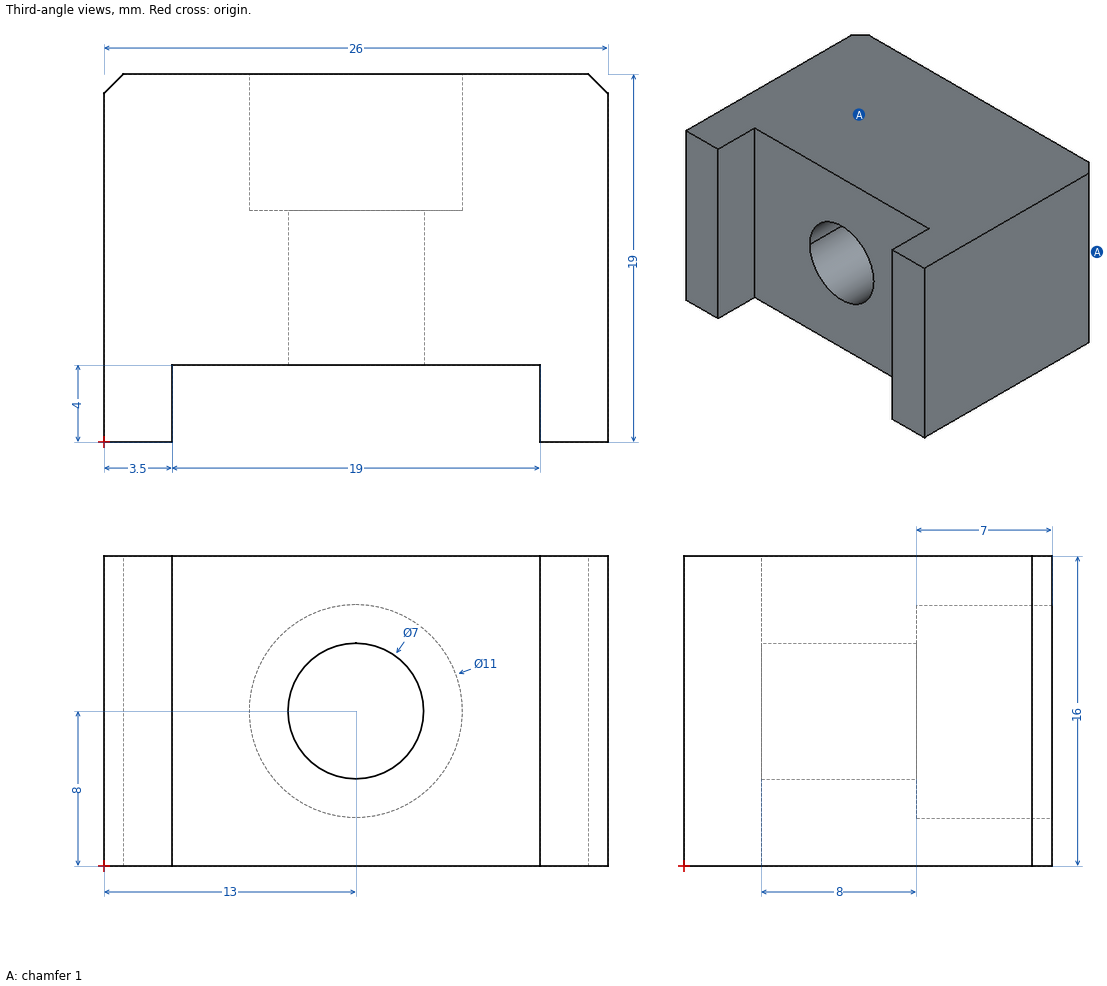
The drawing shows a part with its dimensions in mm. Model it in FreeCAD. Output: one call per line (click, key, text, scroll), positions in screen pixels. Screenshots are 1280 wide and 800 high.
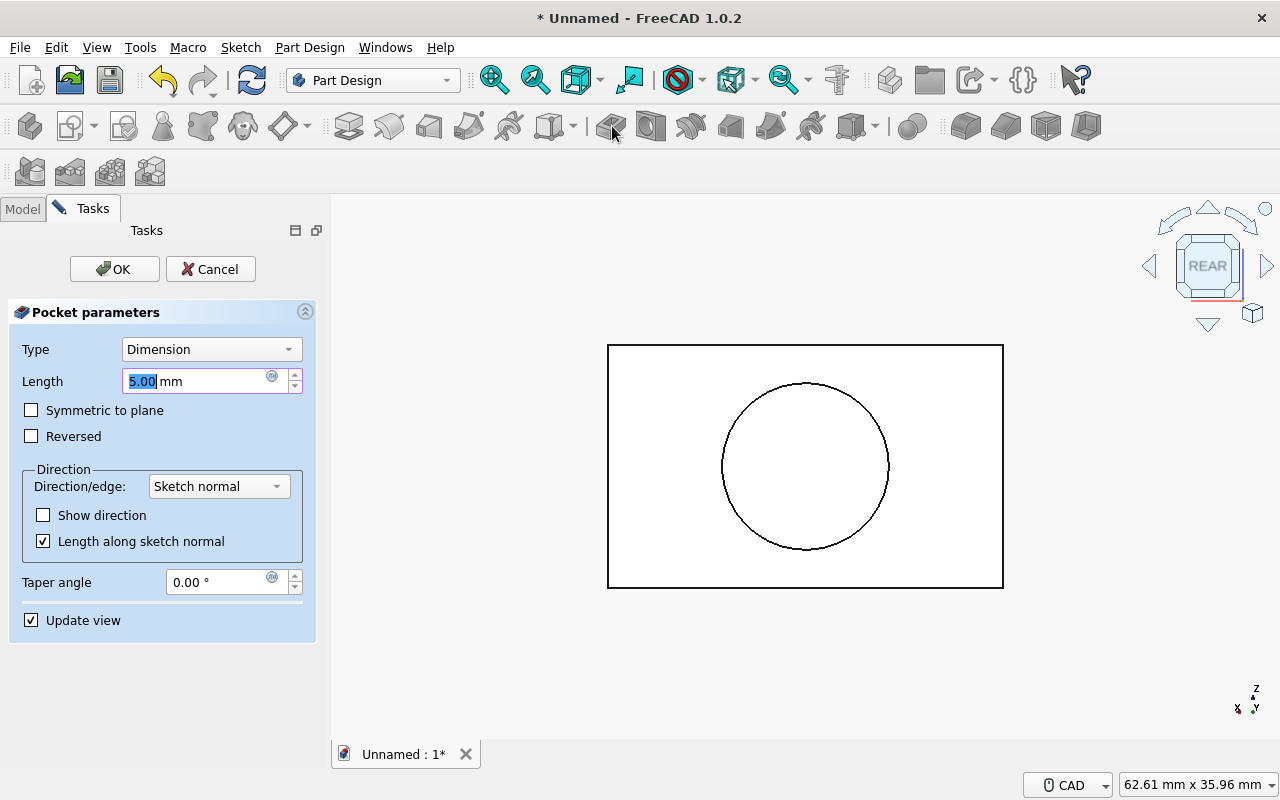
text(7)
key(Tab)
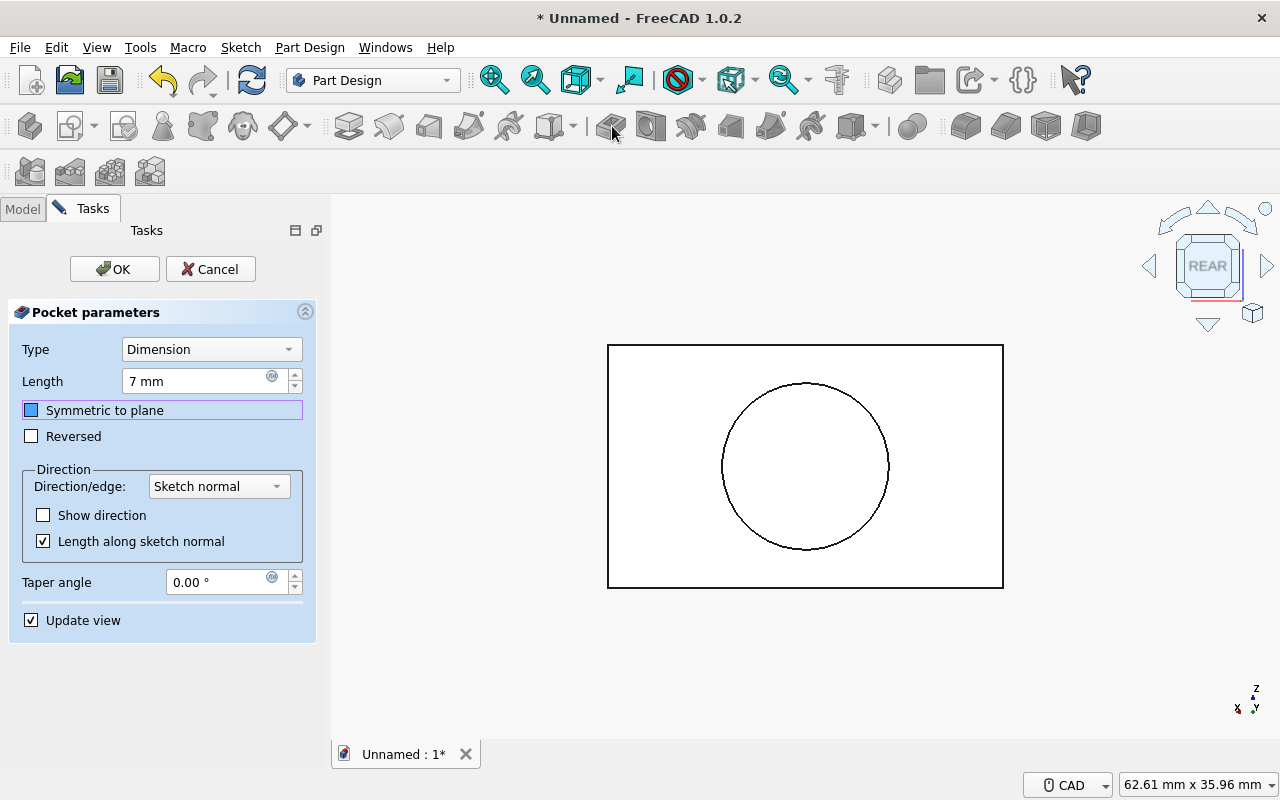
click(115, 269)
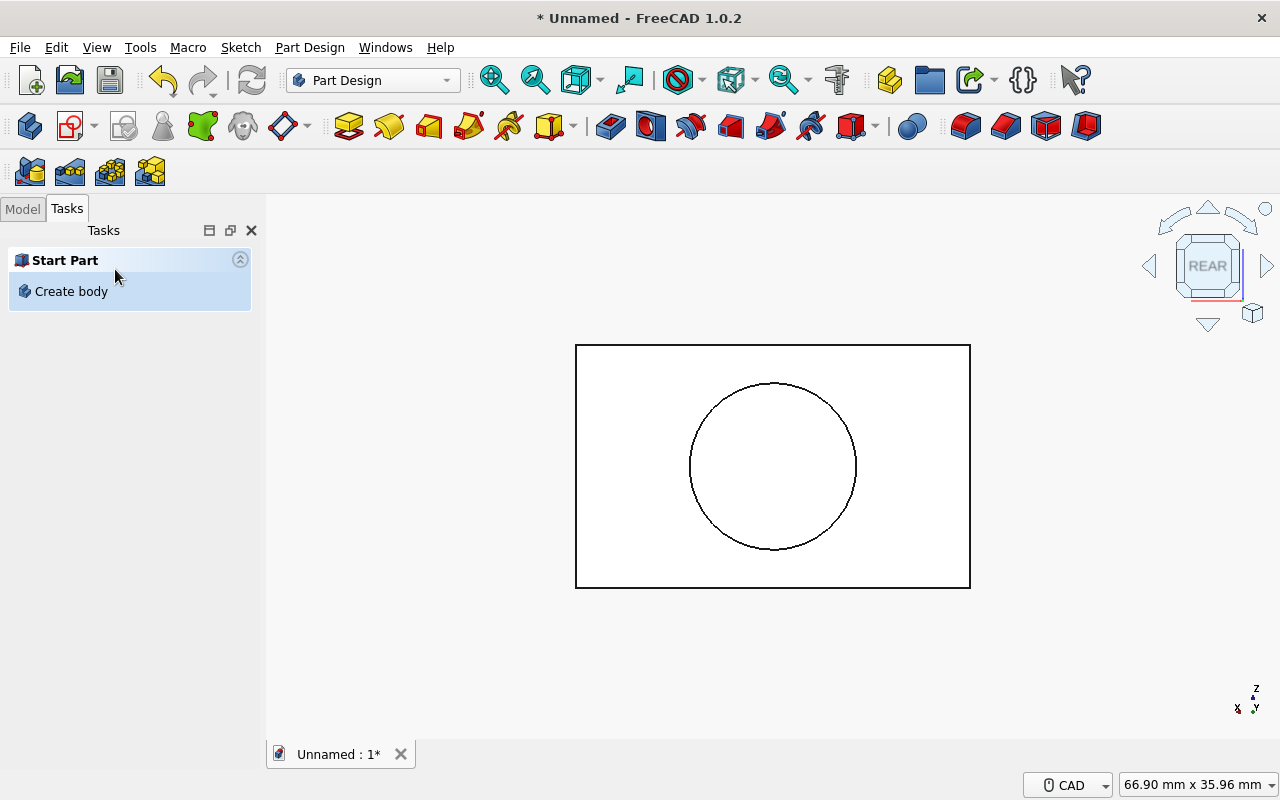
key(v)
key(f)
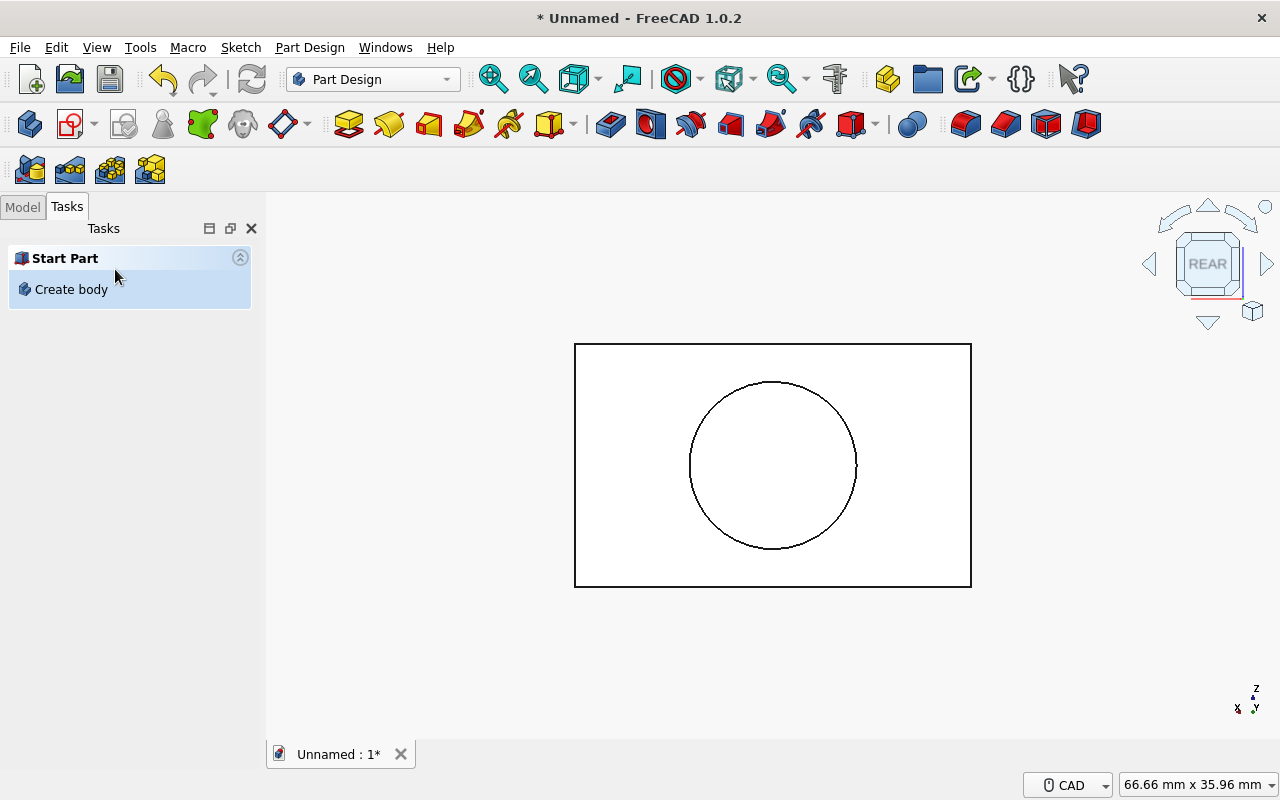
click(773, 464)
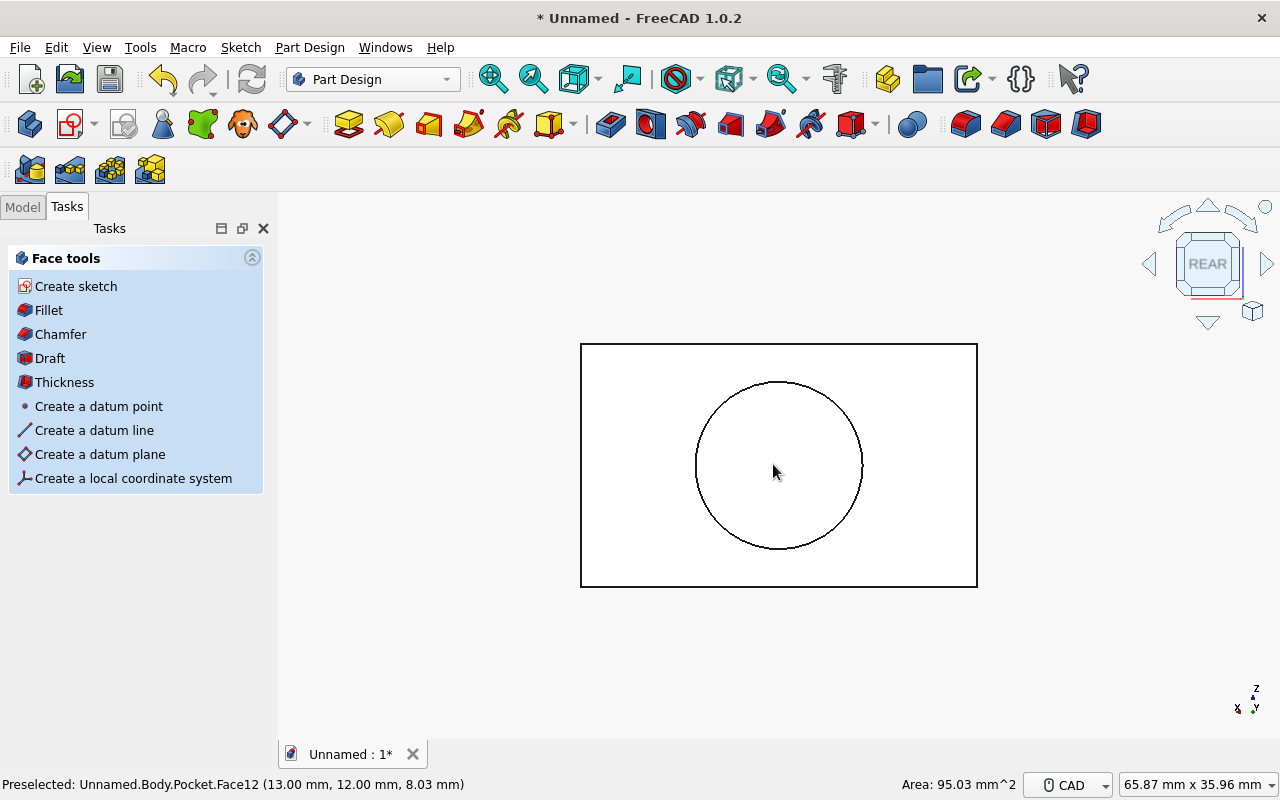
click(70, 124)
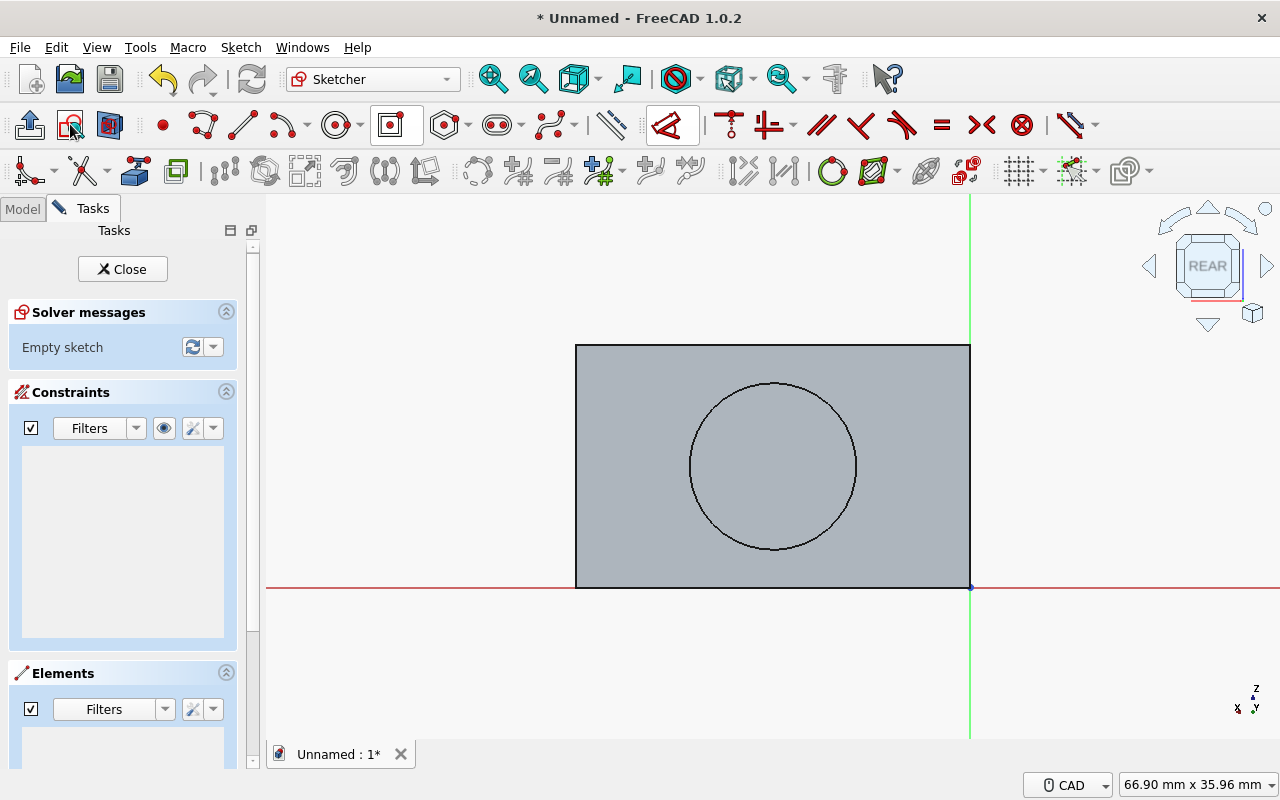
key(q)
key(s)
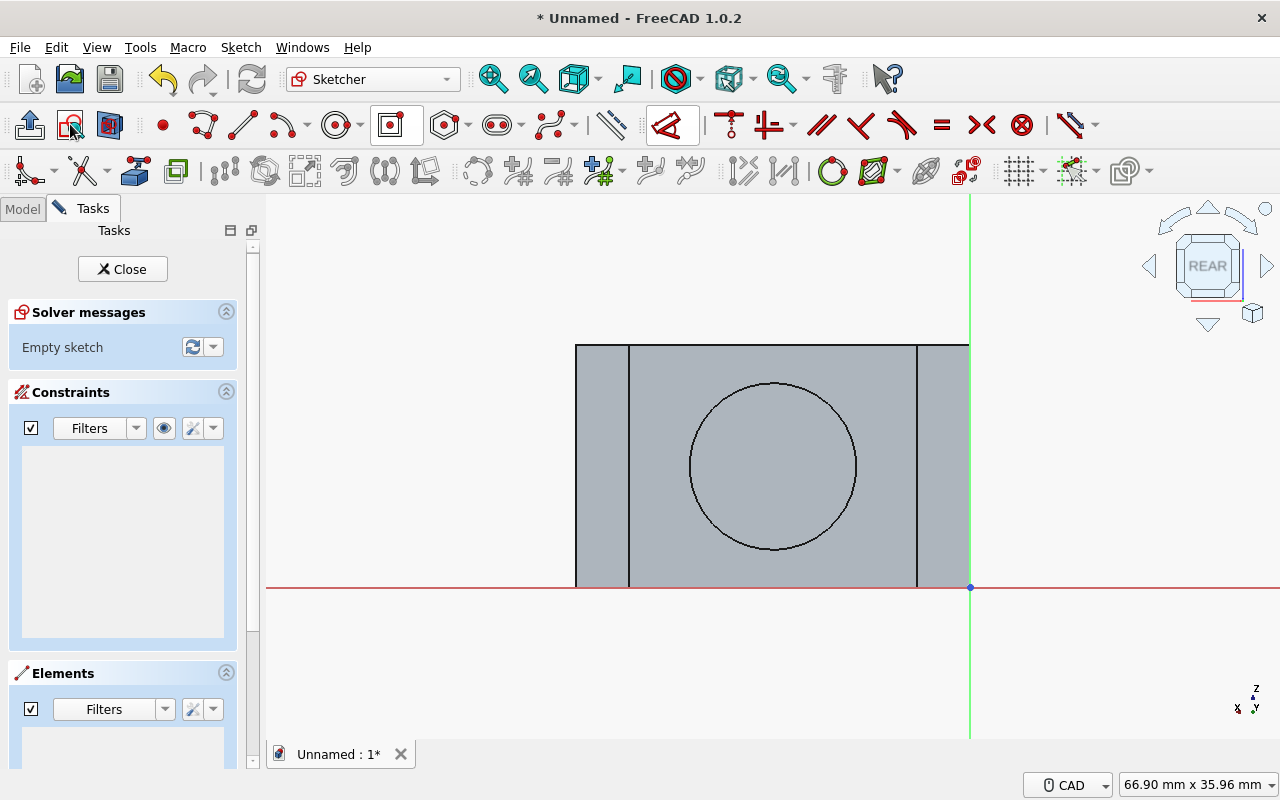
scroll(1016, 542, up, 3)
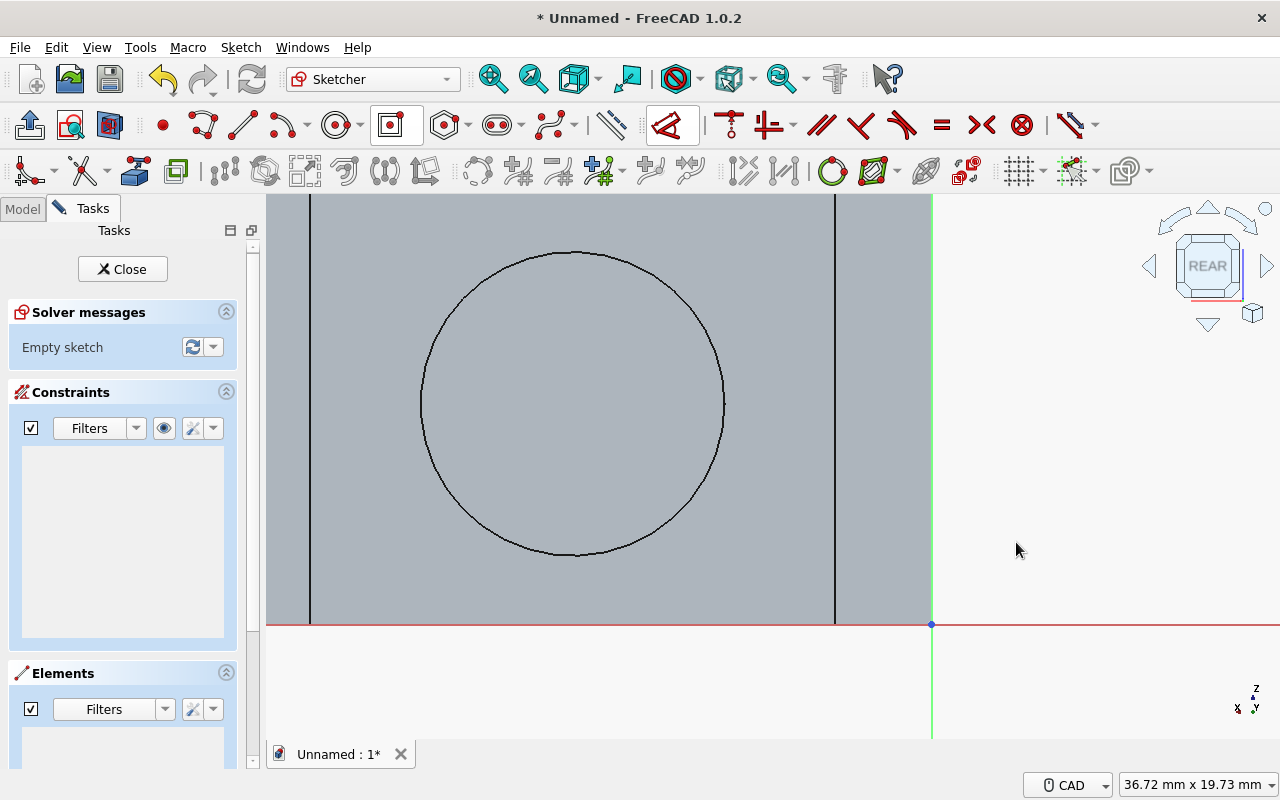
click(336, 126)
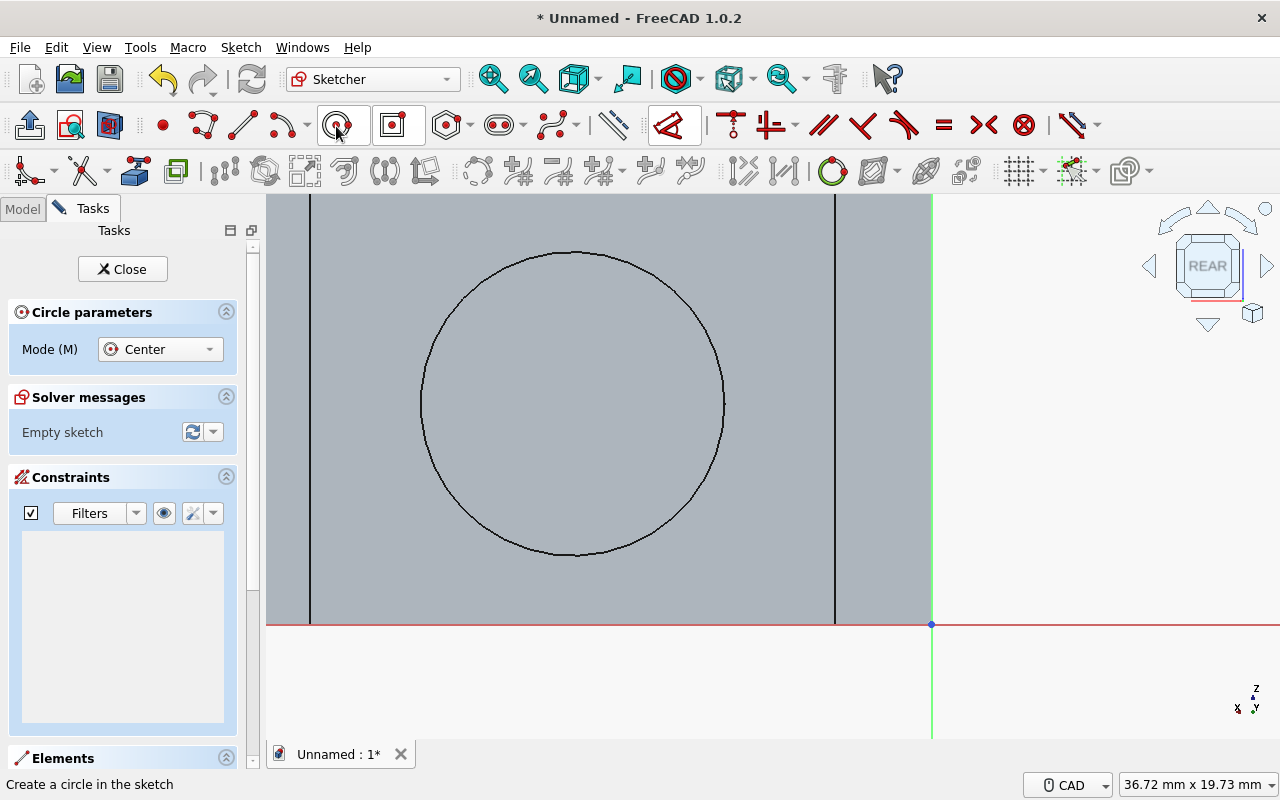
click(573, 404)
move(641, 336)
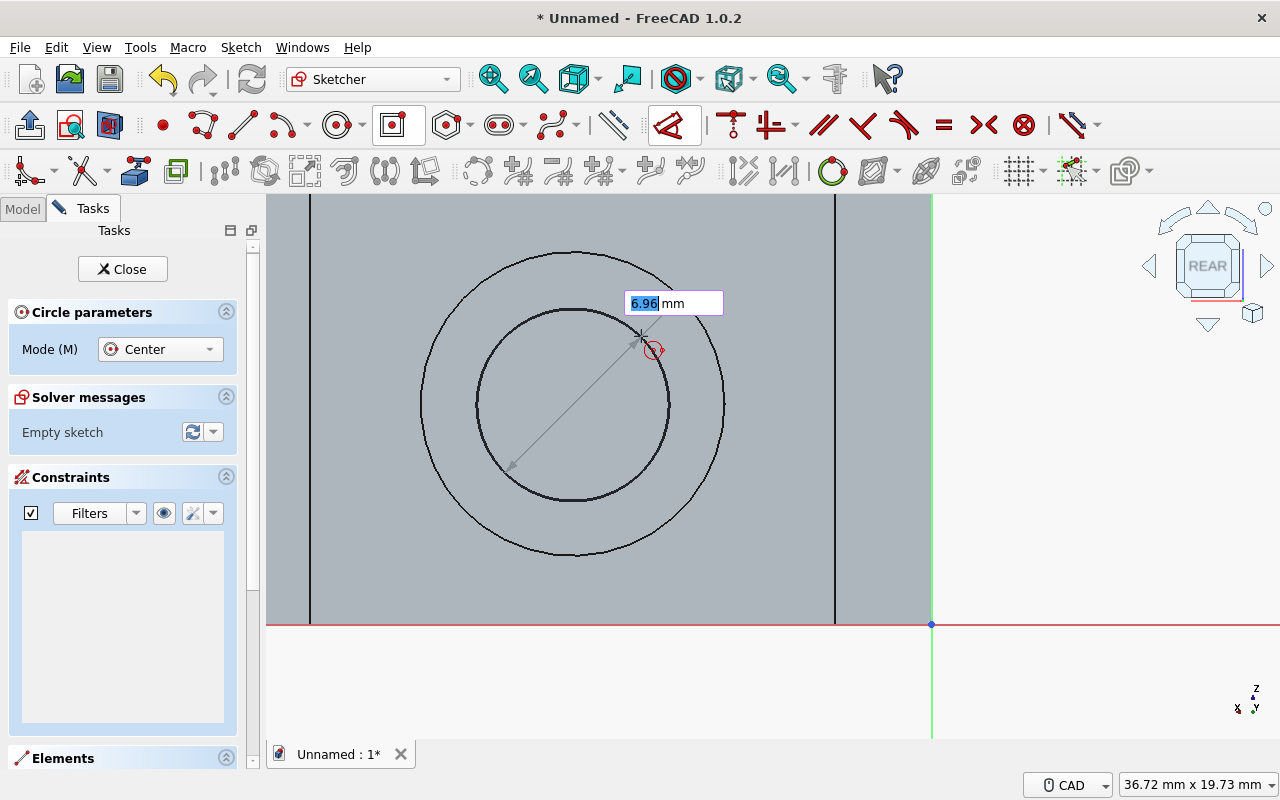
text(7)
key(Return)
key(Escape)